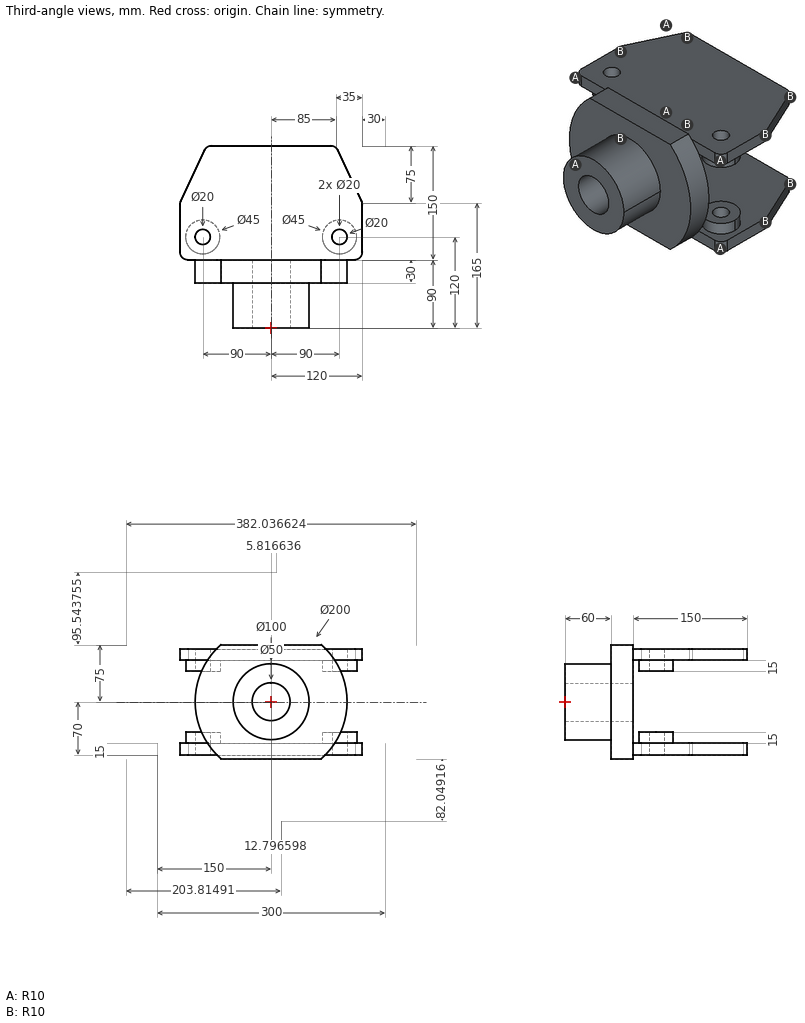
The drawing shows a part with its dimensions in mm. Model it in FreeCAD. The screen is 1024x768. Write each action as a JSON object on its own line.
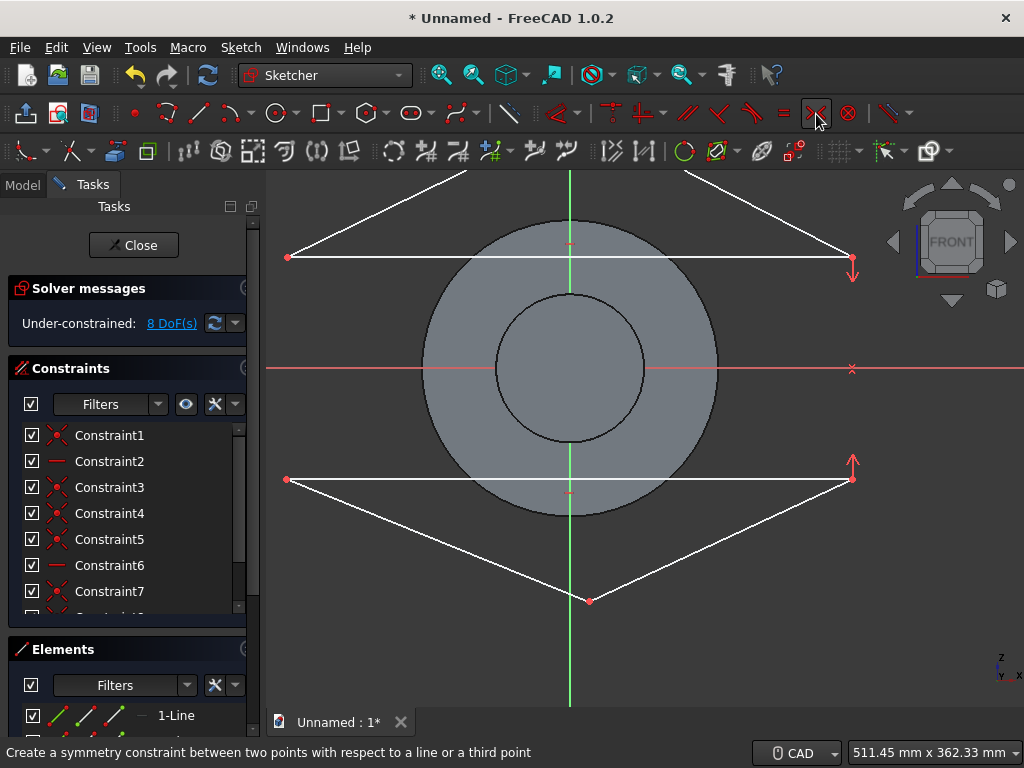
{"action": "left_click", "coordinate": [556, 114]}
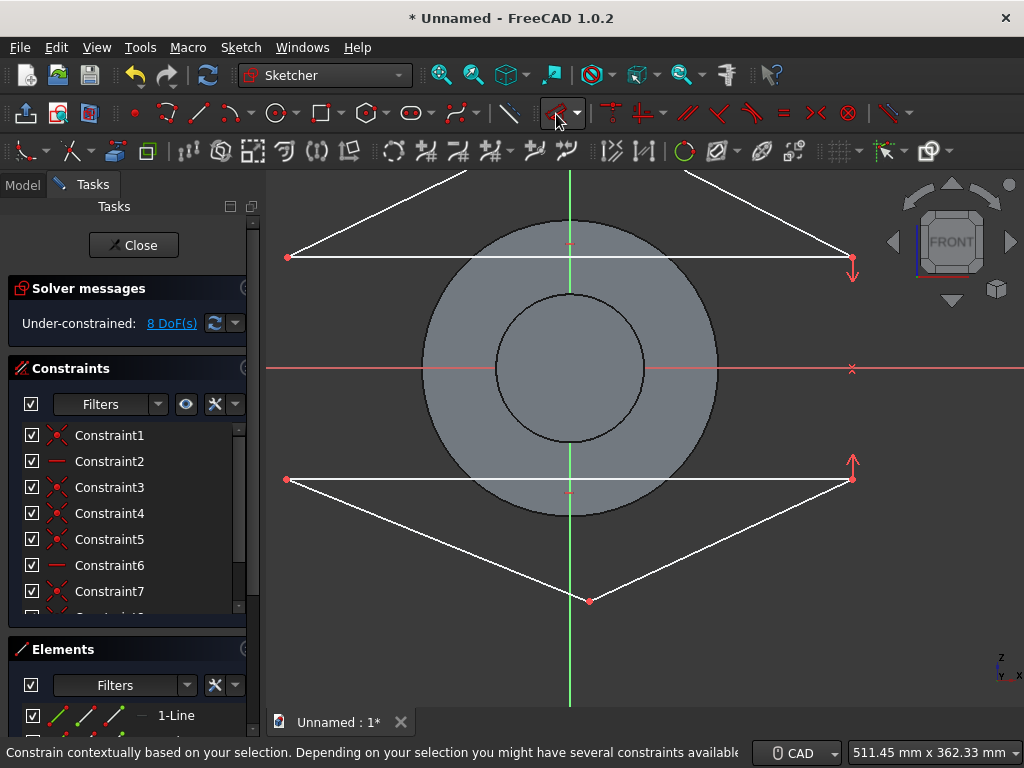
{"action": "scroll", "coordinate": [590, 602], "scroll_direction": "down", "scroll_amount": 2}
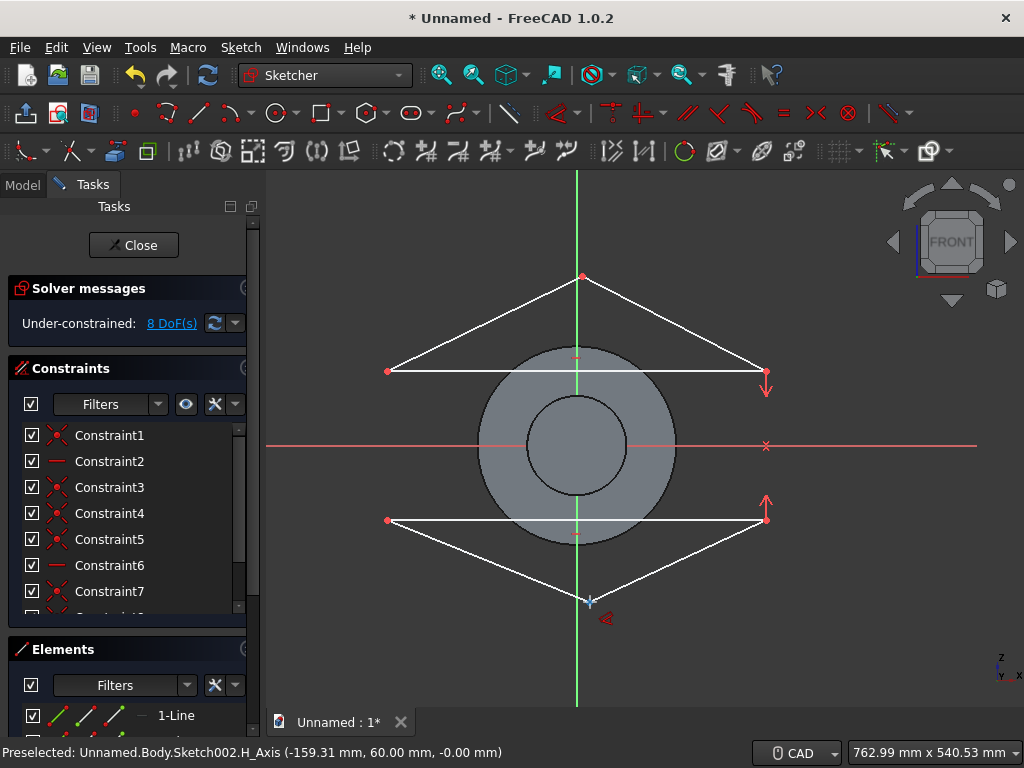
{"action": "left_click", "coordinate": [387, 371]}
{"action": "left_click", "coordinate": [353, 408]}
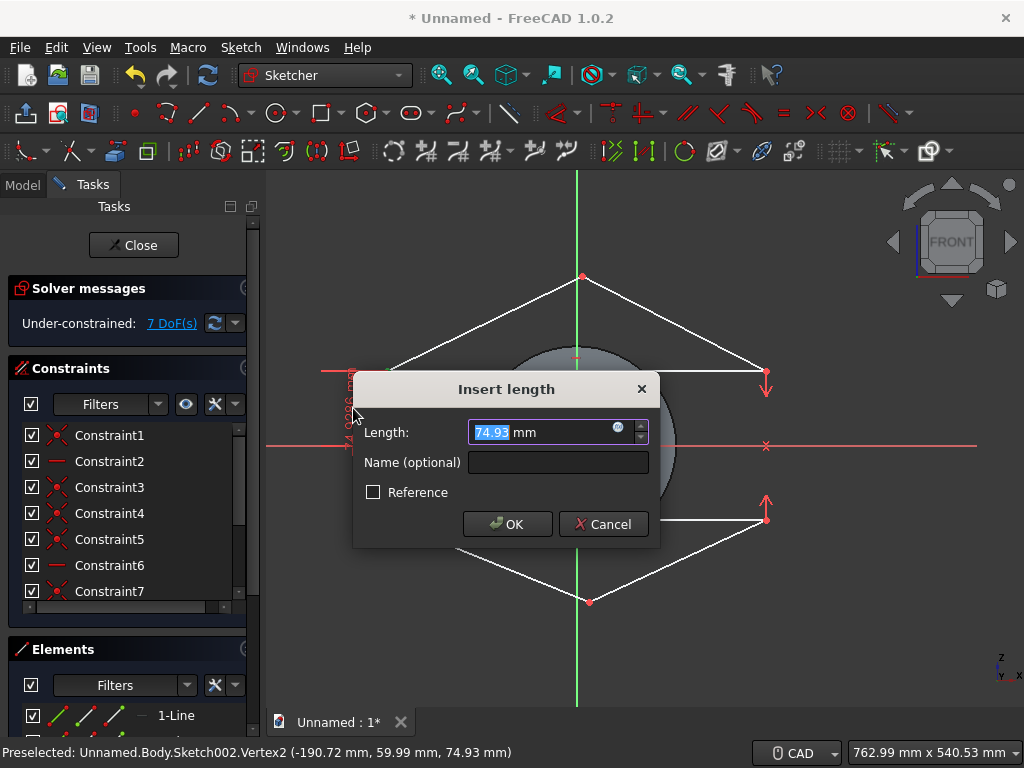
{"action": "type", "text": "75"}
{"action": "key", "text": "Return"}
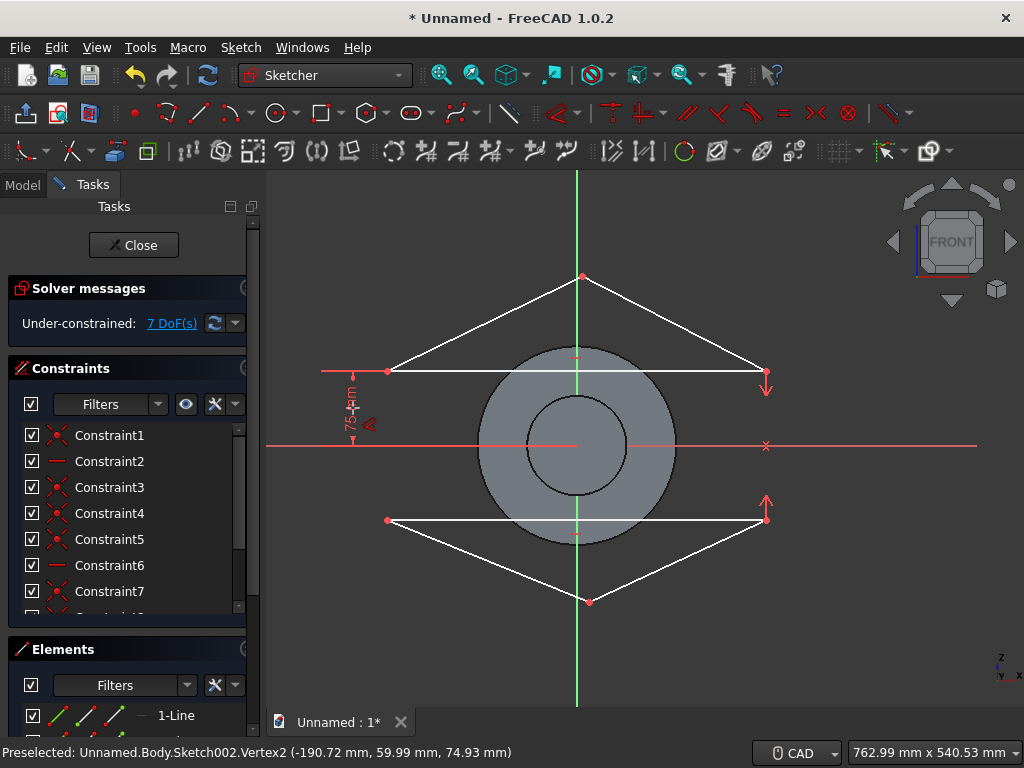
{"action": "scroll", "coordinate": [583, 276], "scroll_direction": "up", "scroll_amount": 10}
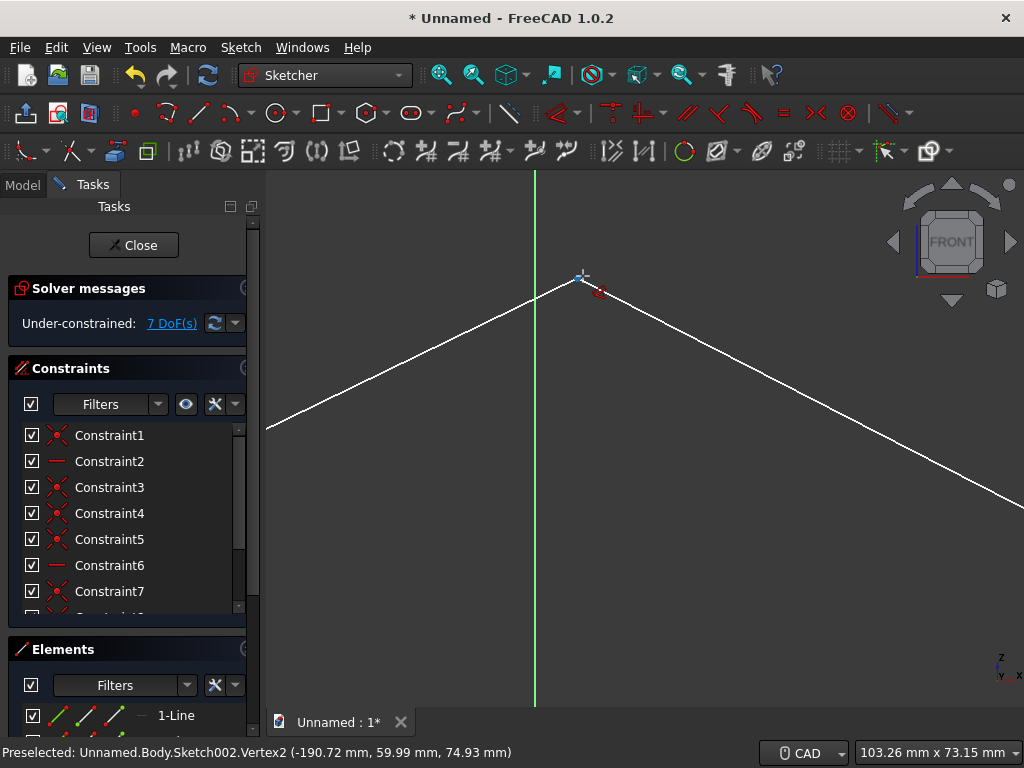
{"action": "left_click", "coordinate": [578, 278]}
{"action": "left_click", "coordinate": [556, 244]}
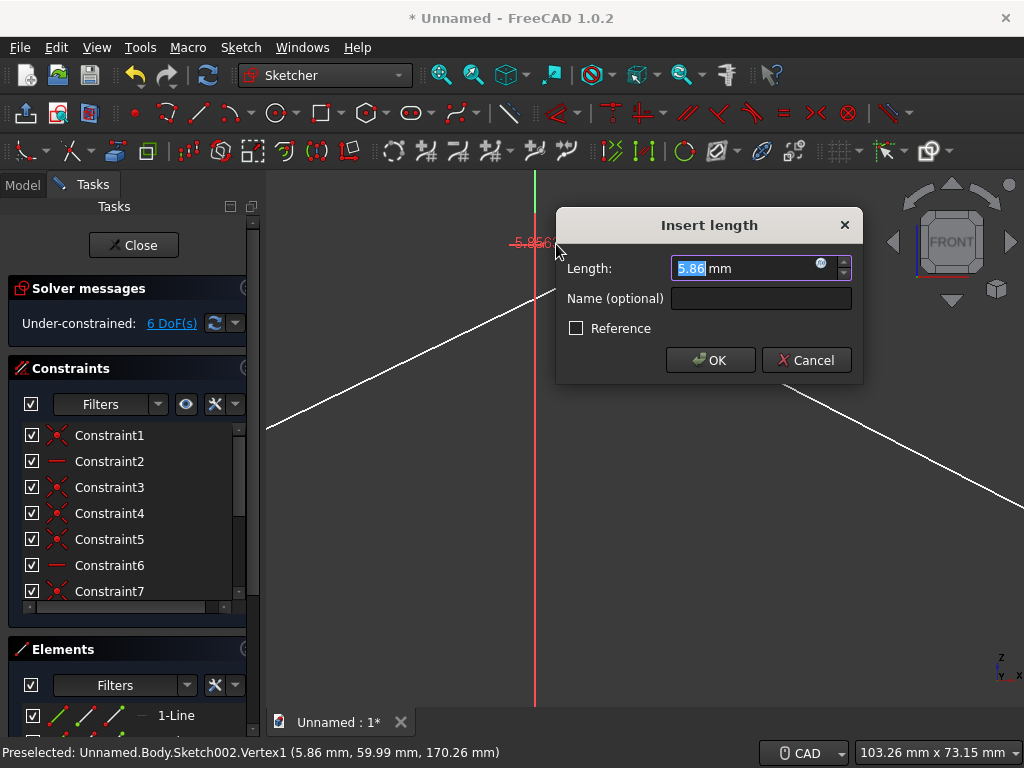
{"action": "type", "text": "5.816636"}
{"action": "key", "text": "Return"}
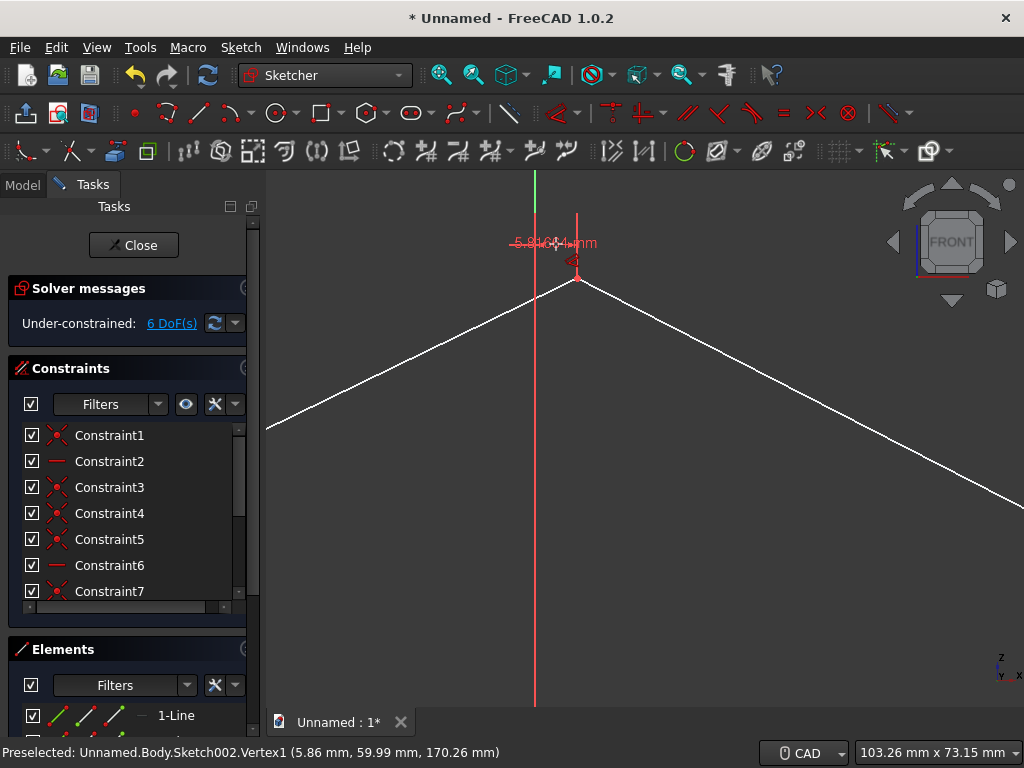
{"action": "scroll", "coordinate": [583, 276], "scroll_direction": "down", "scroll_amount": 10}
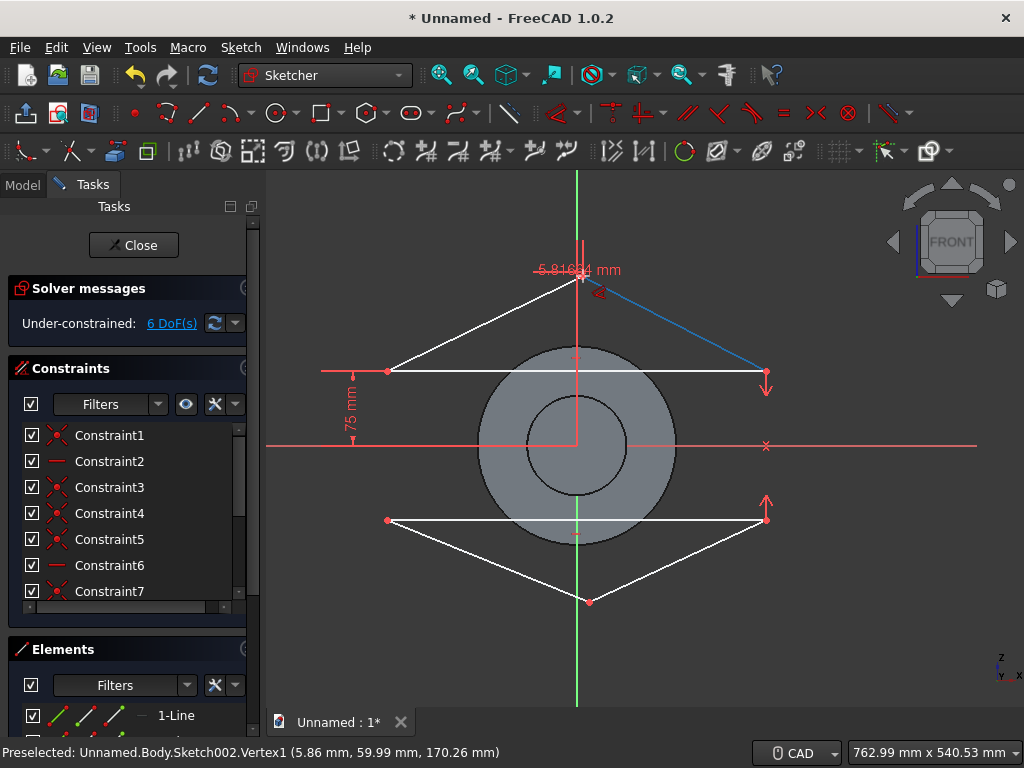
{"action": "left_click", "coordinate": [643, 578]}
{"action": "left_click", "coordinate": [800, 561]}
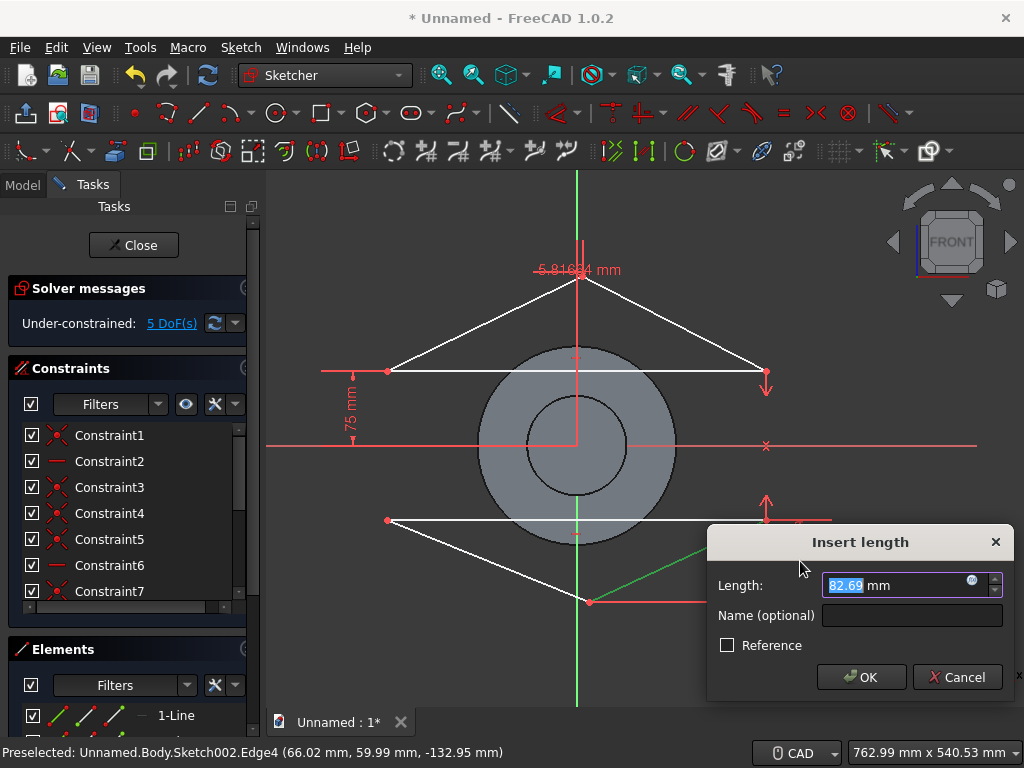
{"action": "type", "text": "82.04916"}
{"action": "key", "text": "Return"}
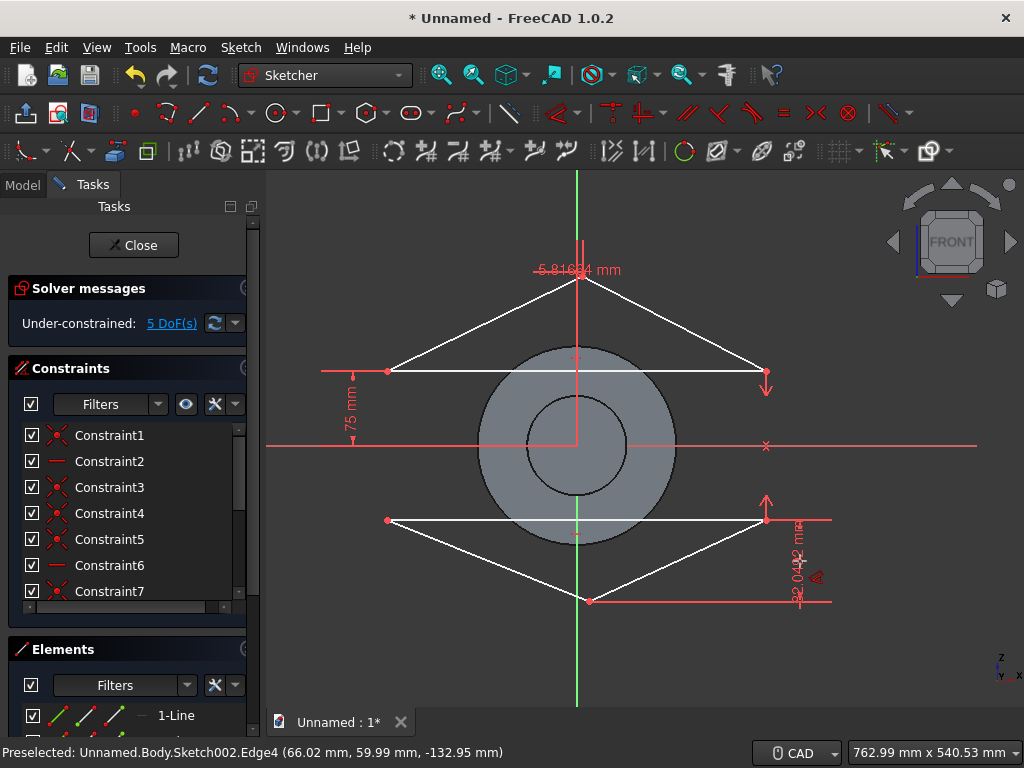
{"action": "left_click", "coordinate": [501, 371]}
{"action": "left_click", "coordinate": [490, 337]}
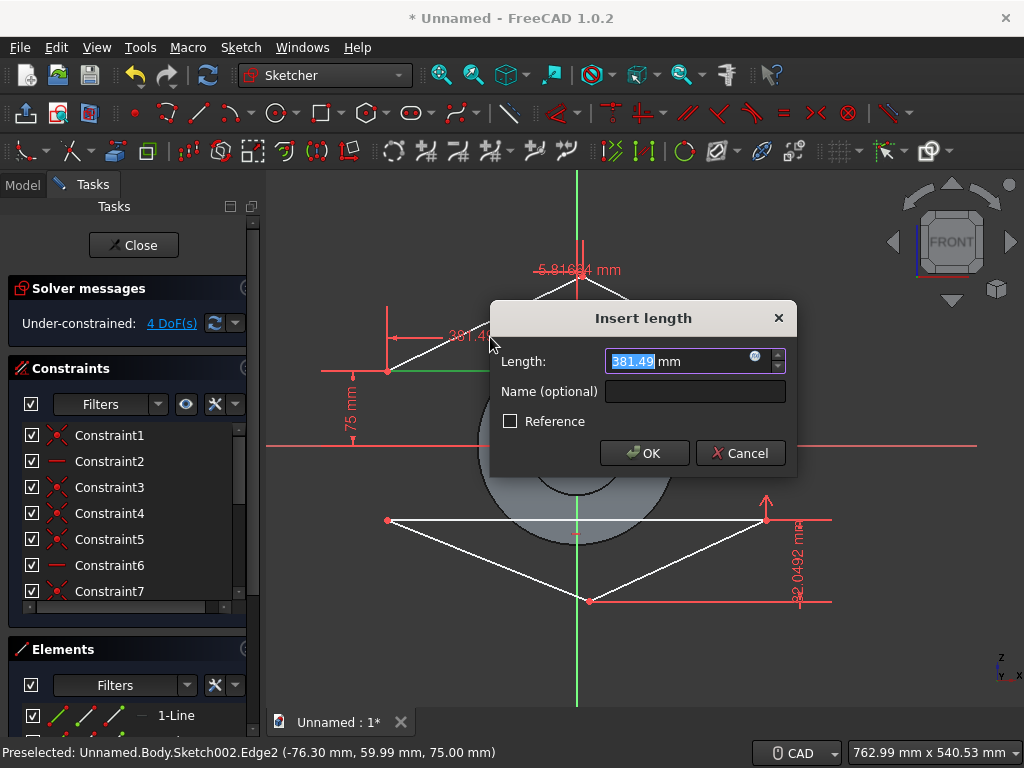
{"action": "type", "text": "382.036624"}
{"action": "key", "text": "Return"}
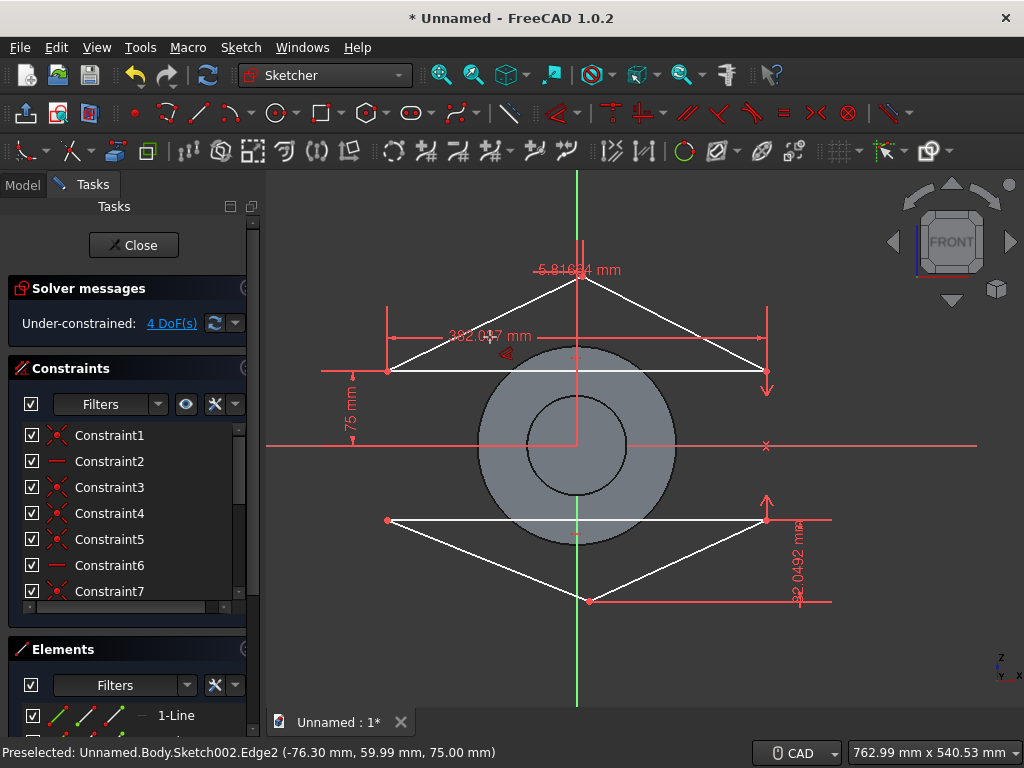
{"action": "left_click", "coordinate": [653, 520]}
{"action": "left_click", "coordinate": [490, 486]}